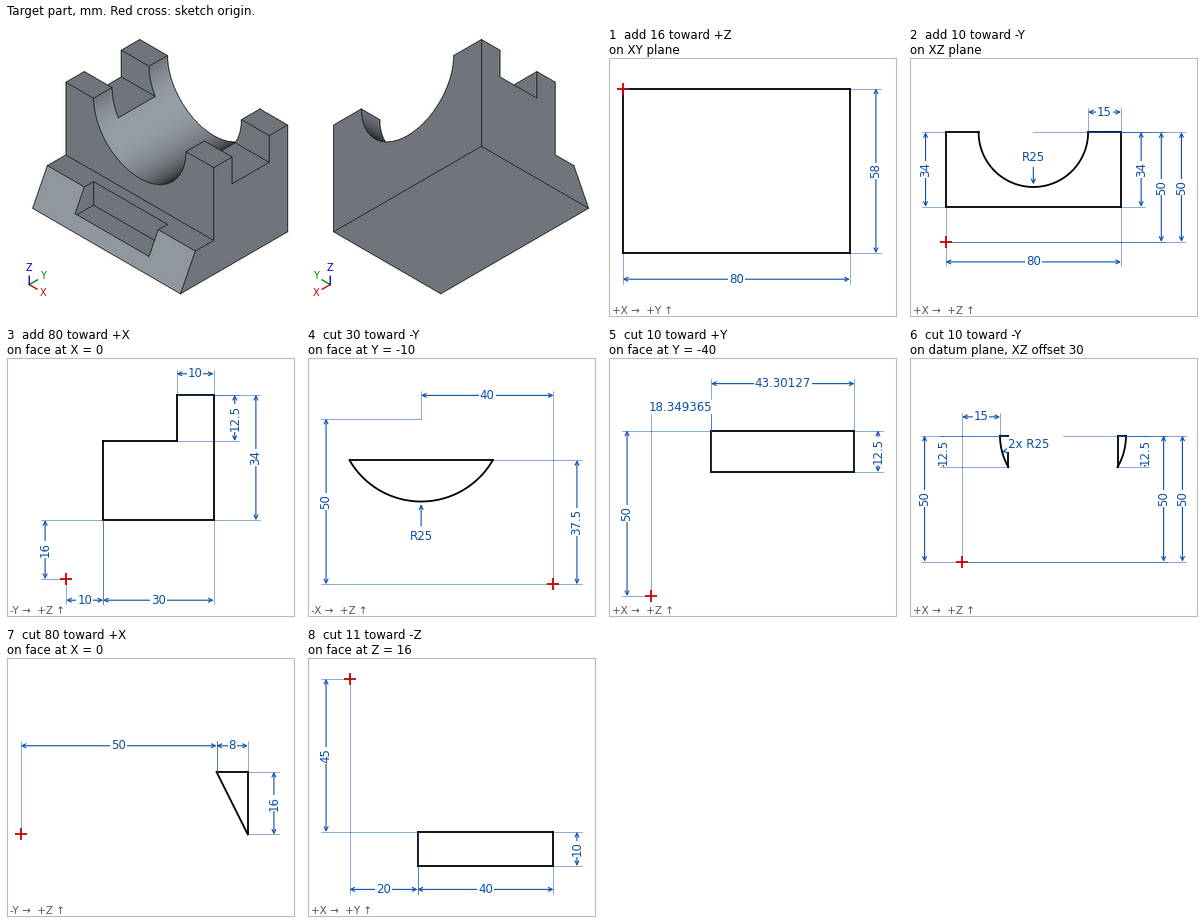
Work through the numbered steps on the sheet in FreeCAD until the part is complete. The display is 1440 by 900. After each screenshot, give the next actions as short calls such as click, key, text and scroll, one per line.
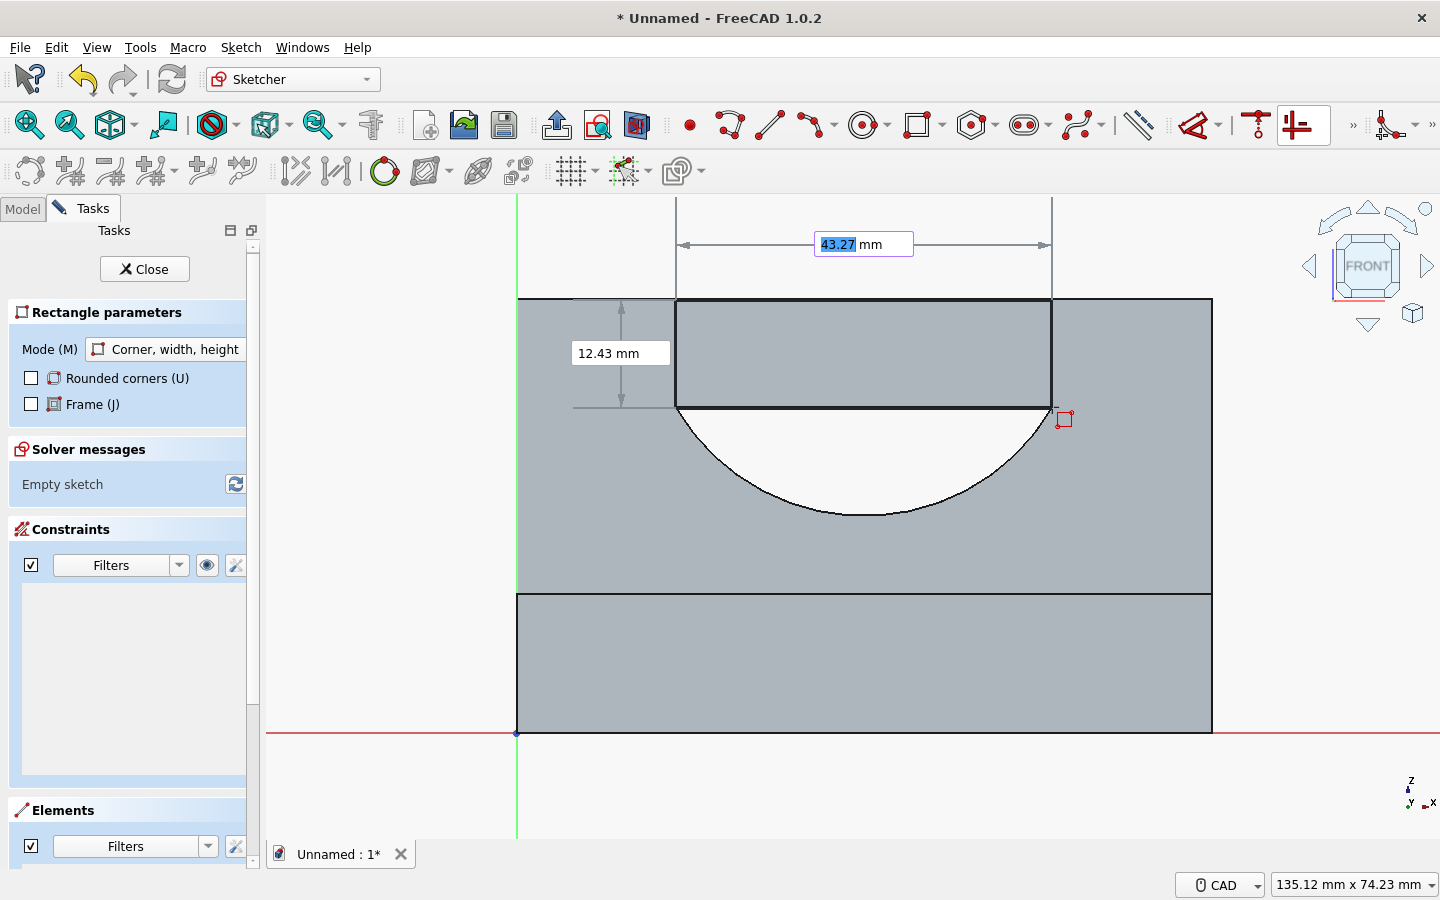
text(43.30127)
key(Tab)
text(12.5)
key(Return)
key(Escape)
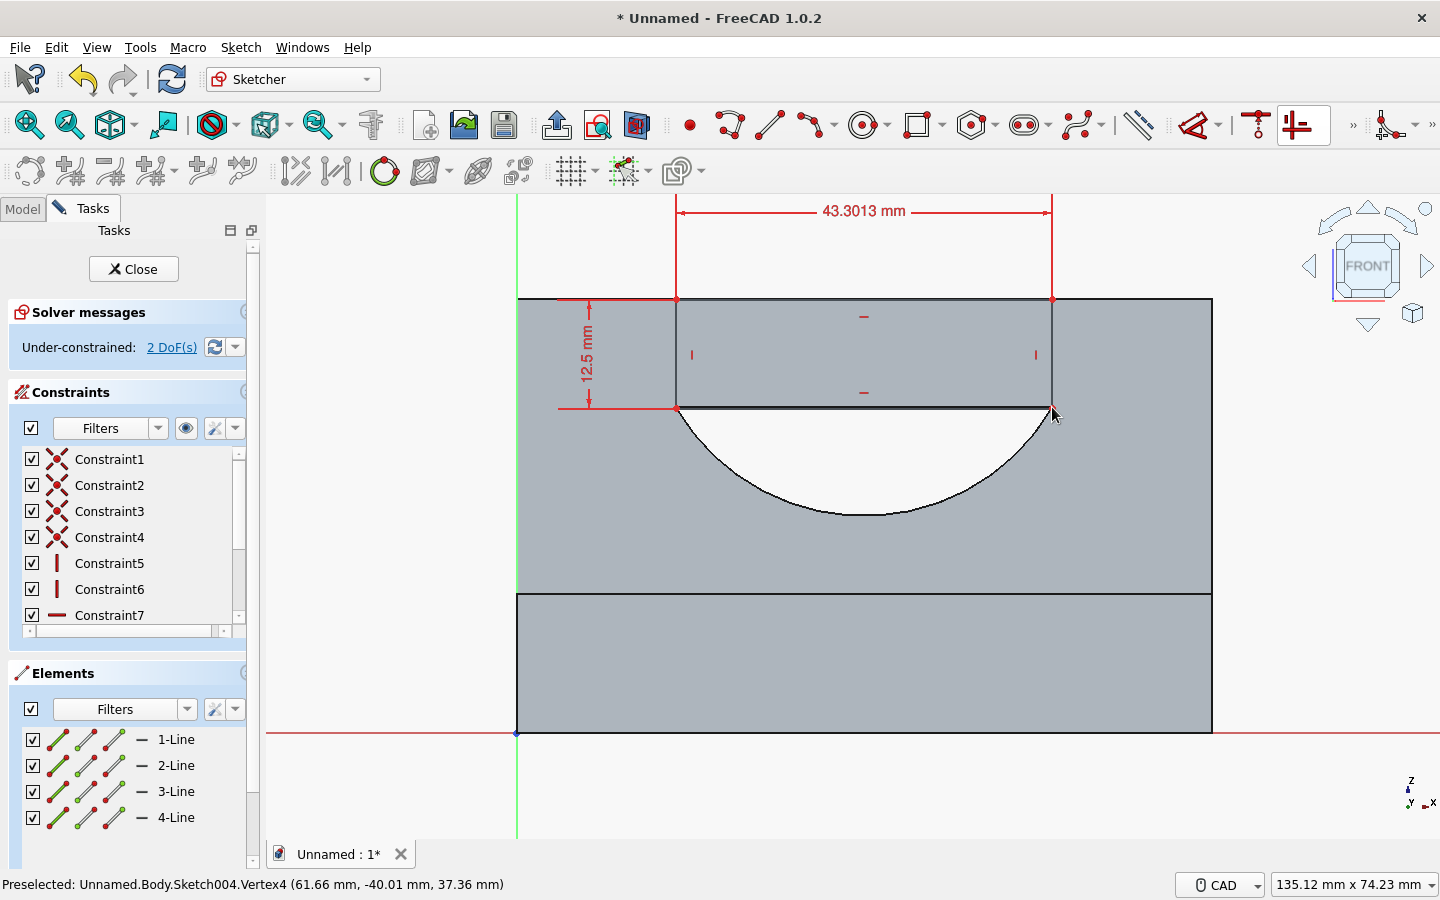
click(1194, 126)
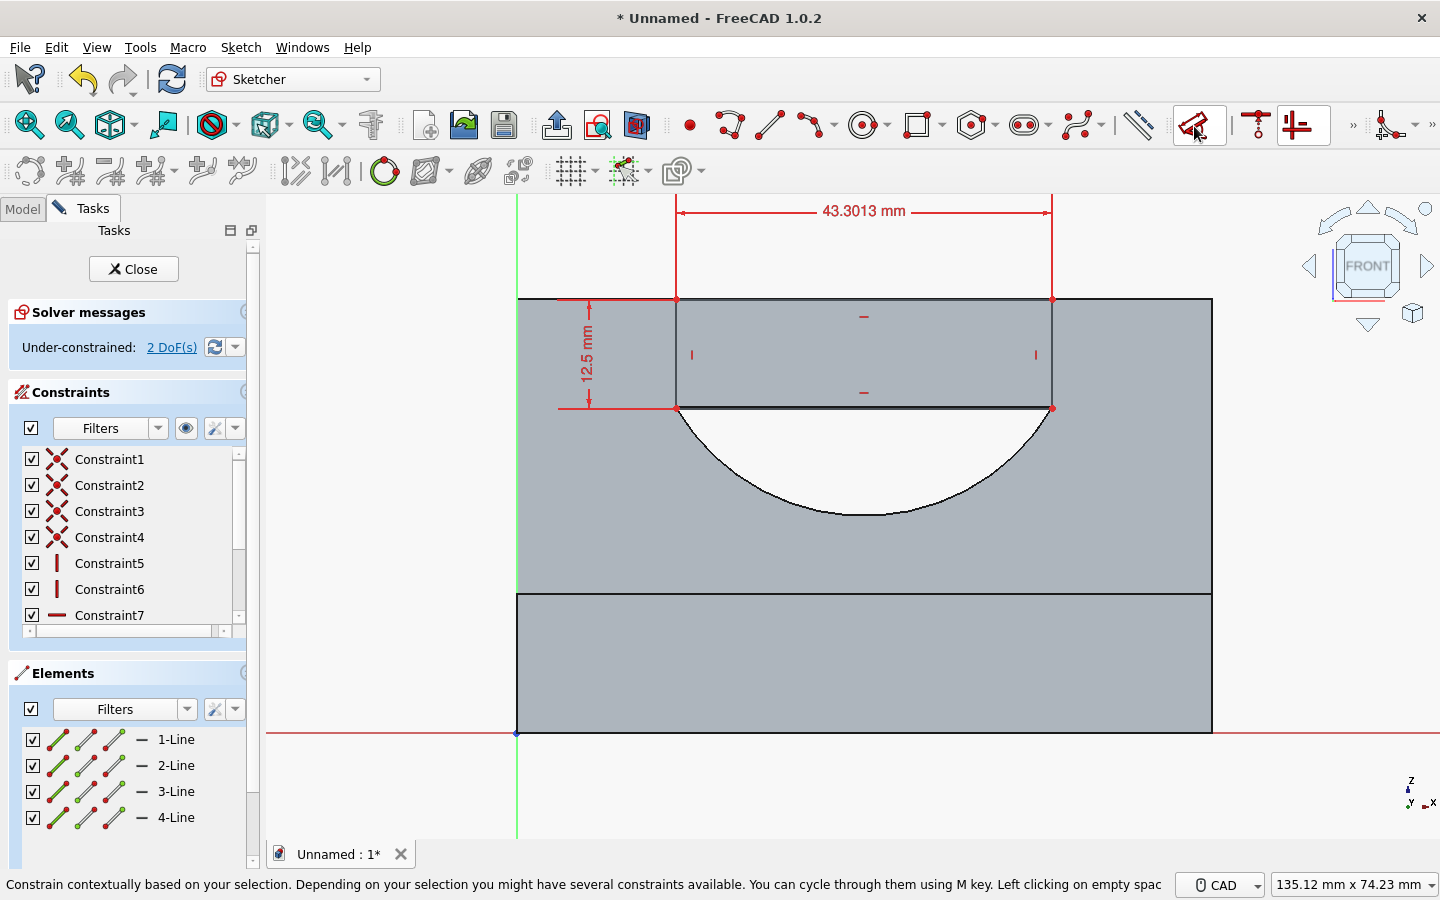
click(676, 300)
click(483, 517)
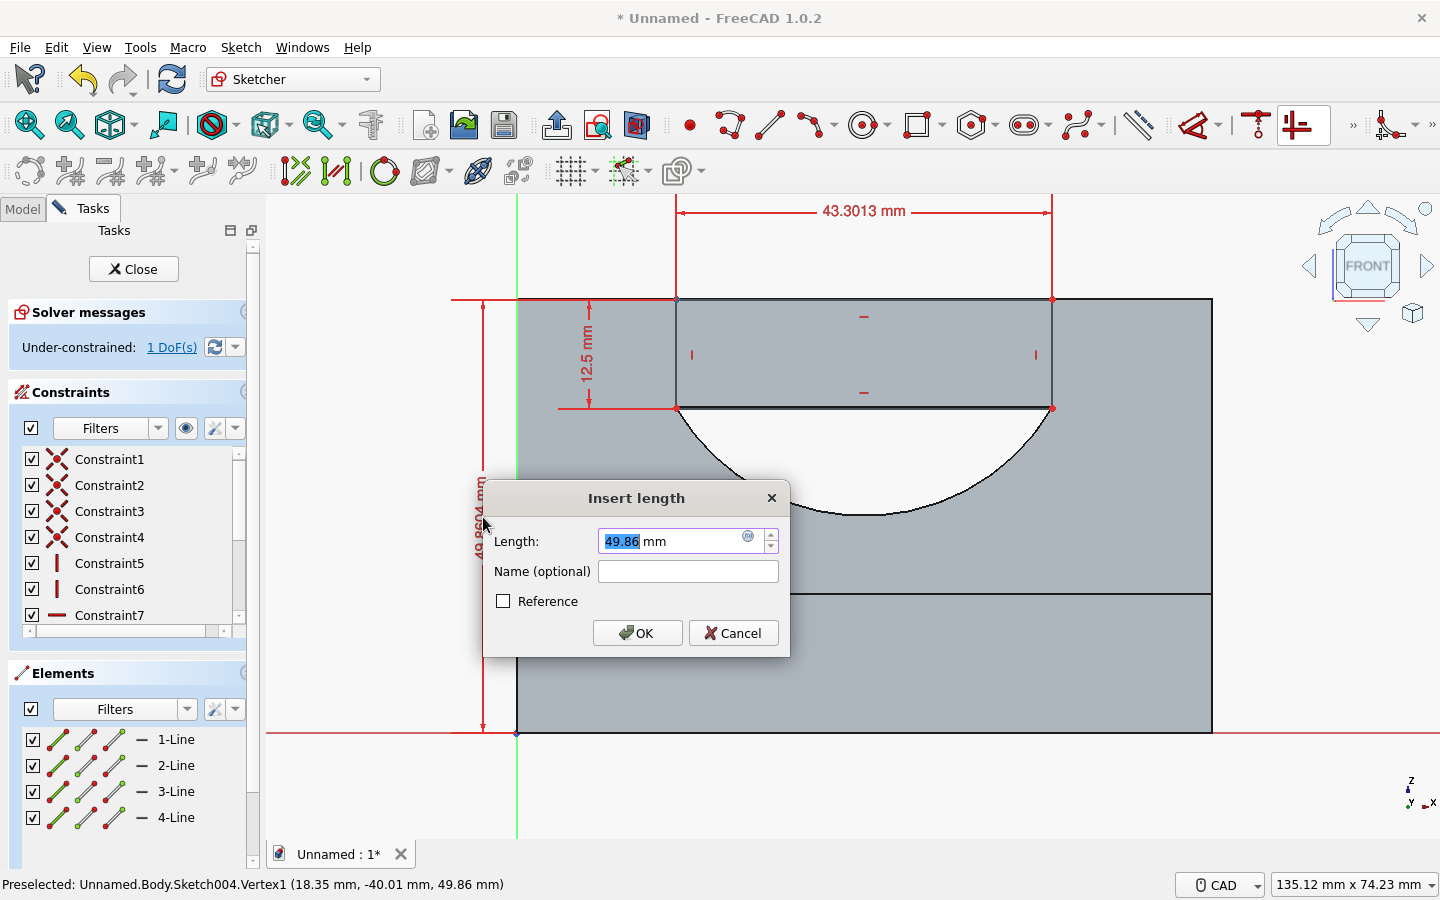
text(50)
key(Return)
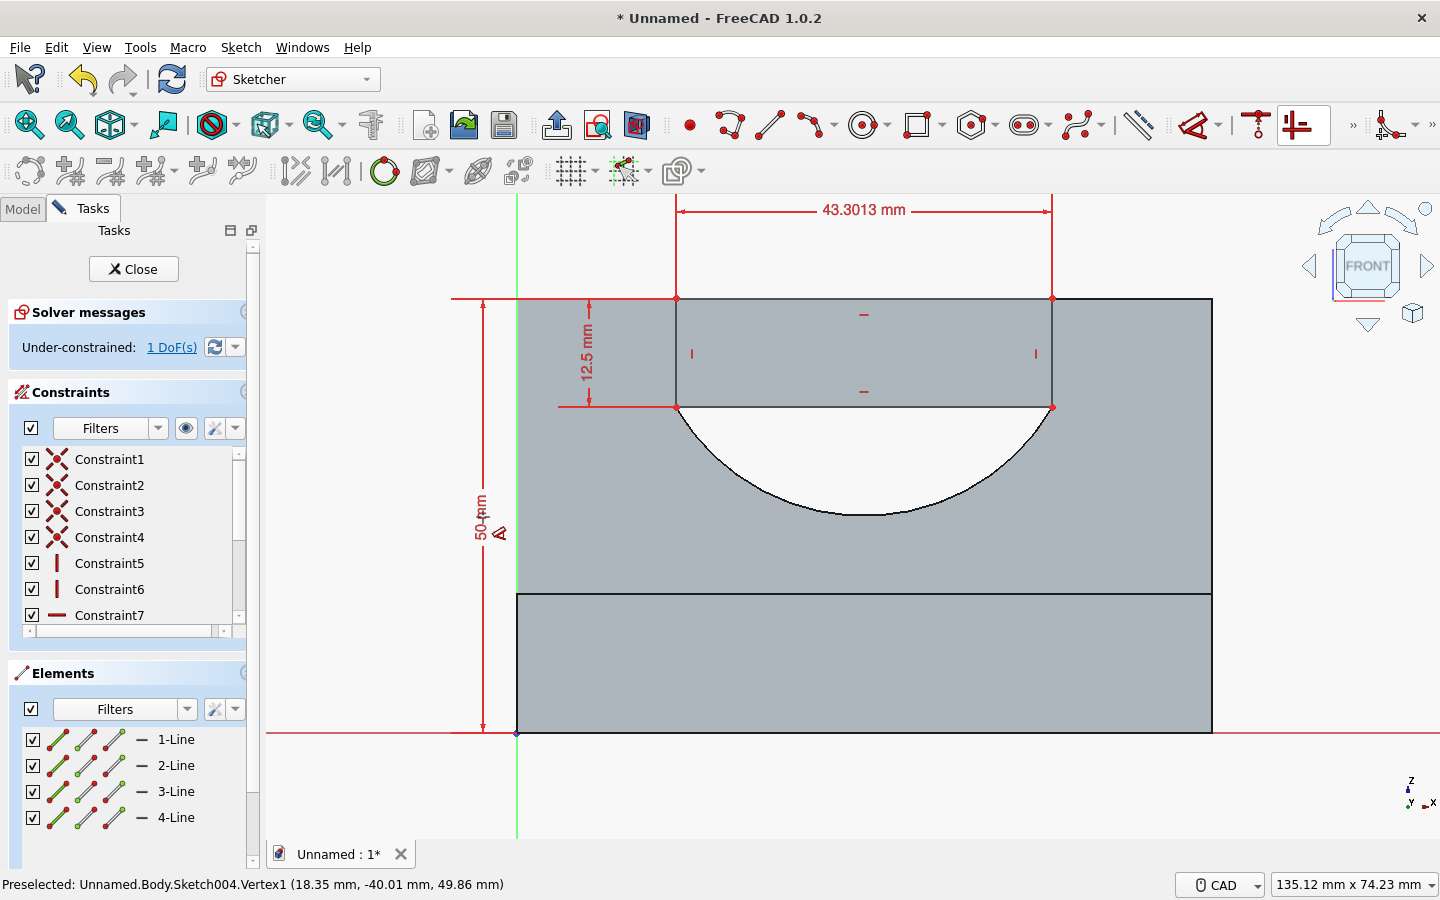
click(676, 299)
click(596, 767)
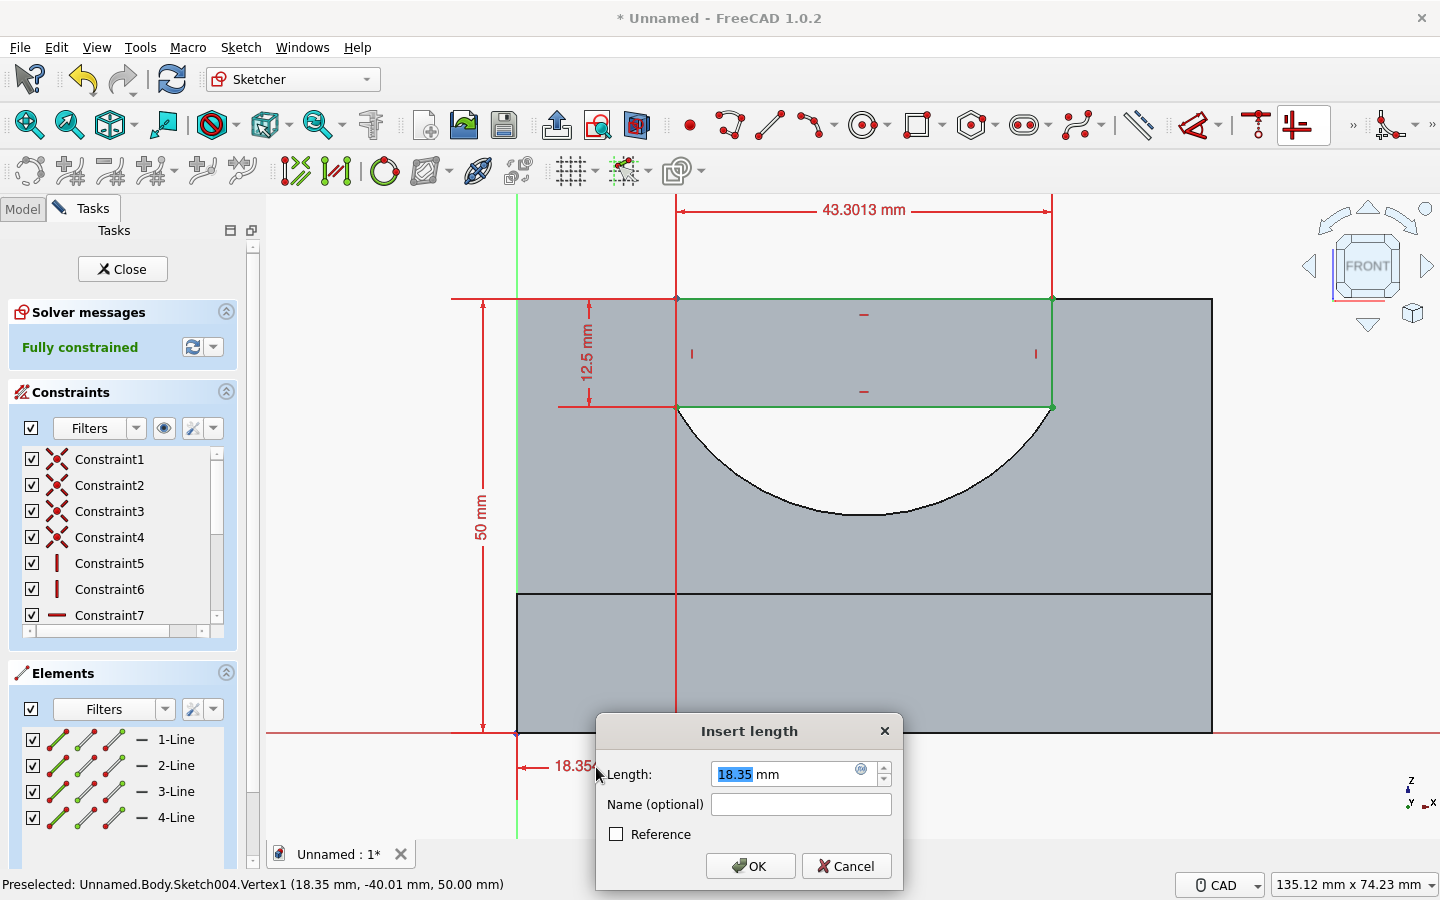
text(18.349365)
key(Return)
key(Escape)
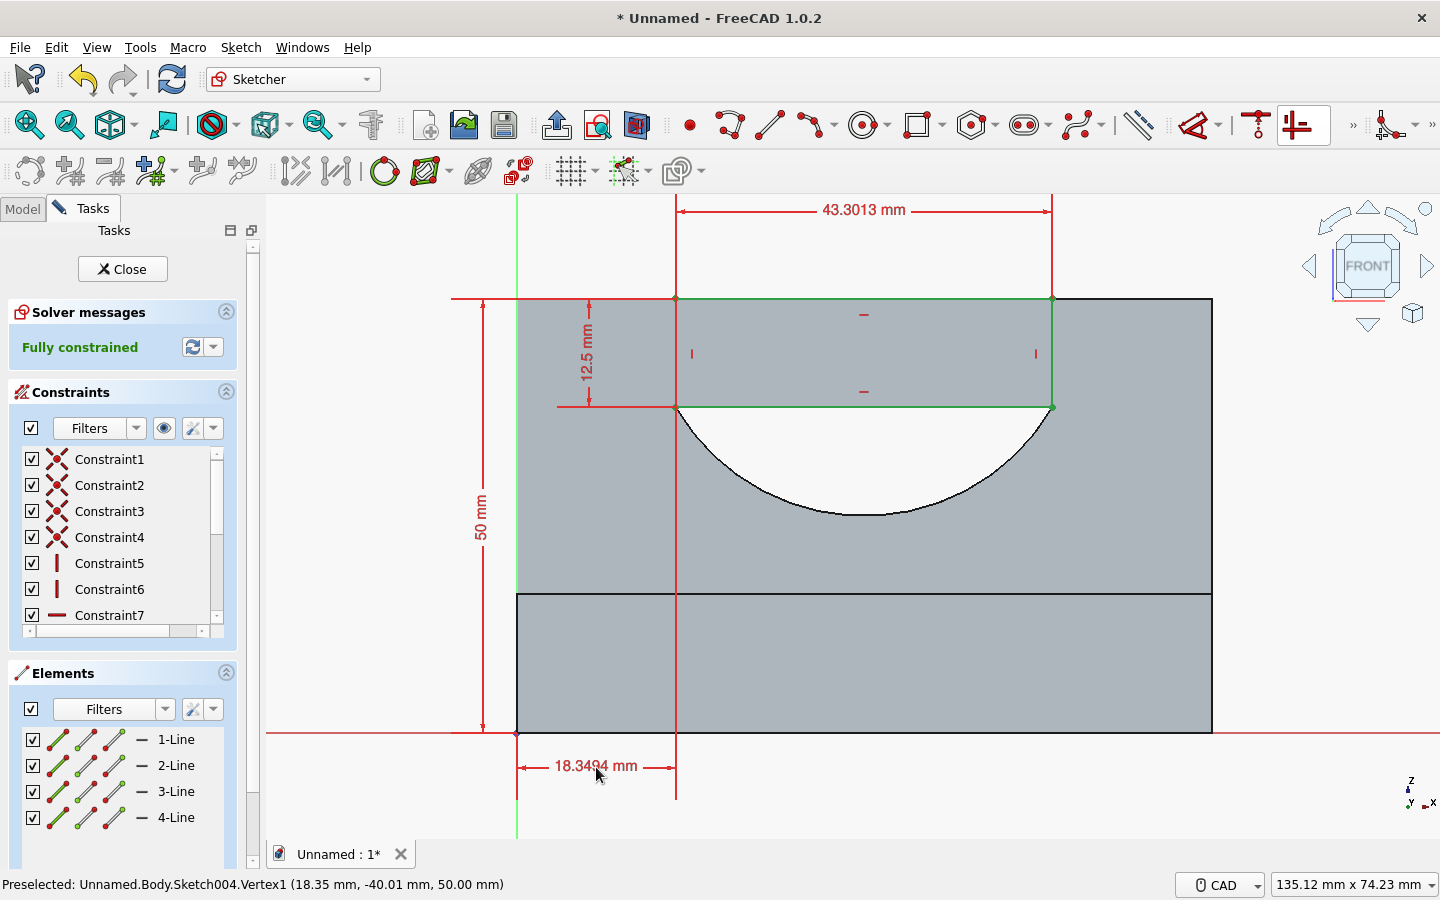
click(123, 269)